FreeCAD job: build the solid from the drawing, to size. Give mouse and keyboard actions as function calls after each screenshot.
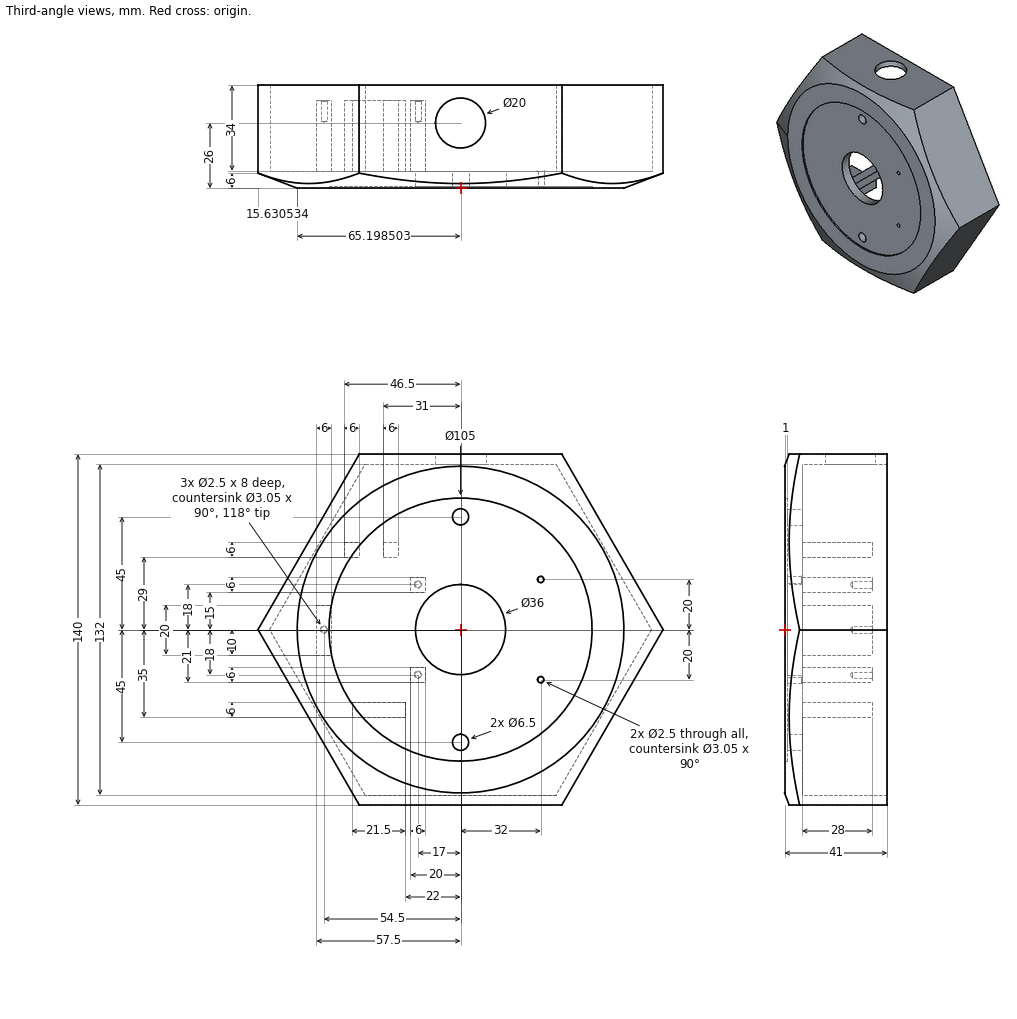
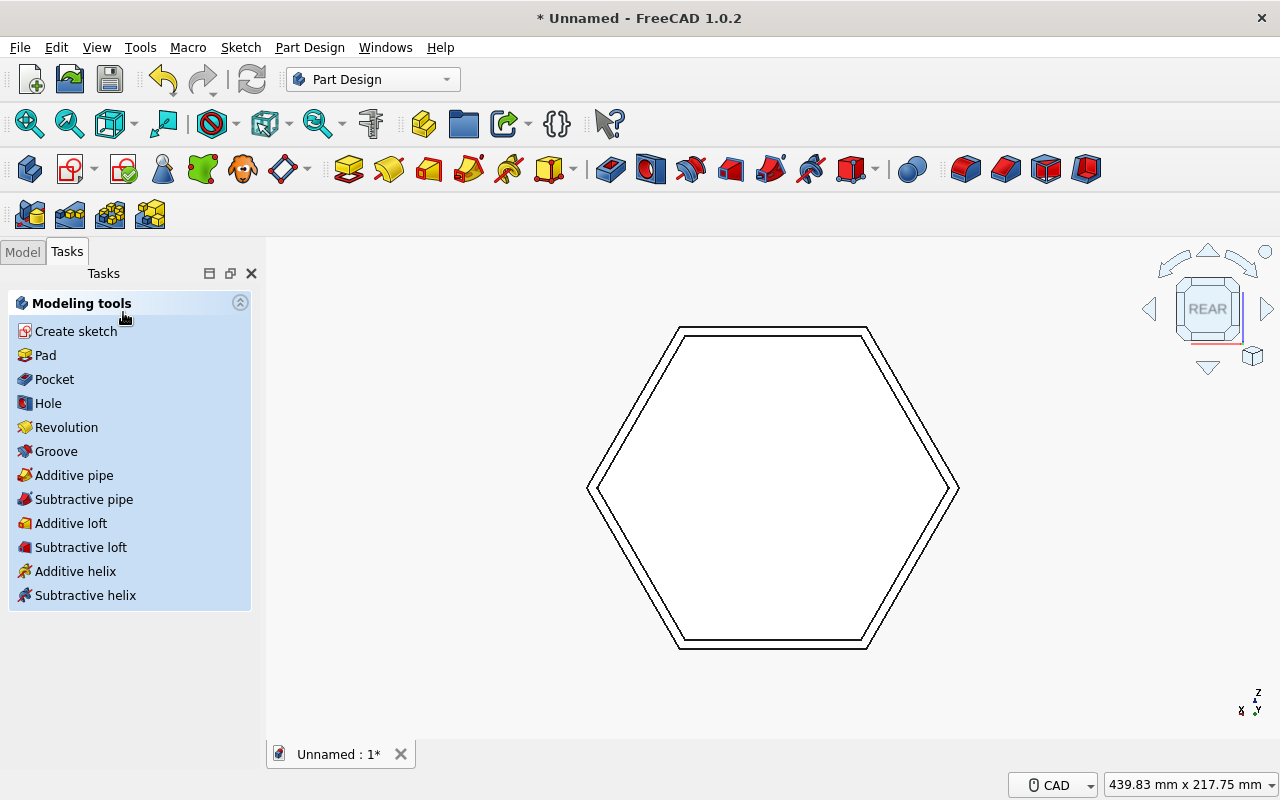
click(612, 170)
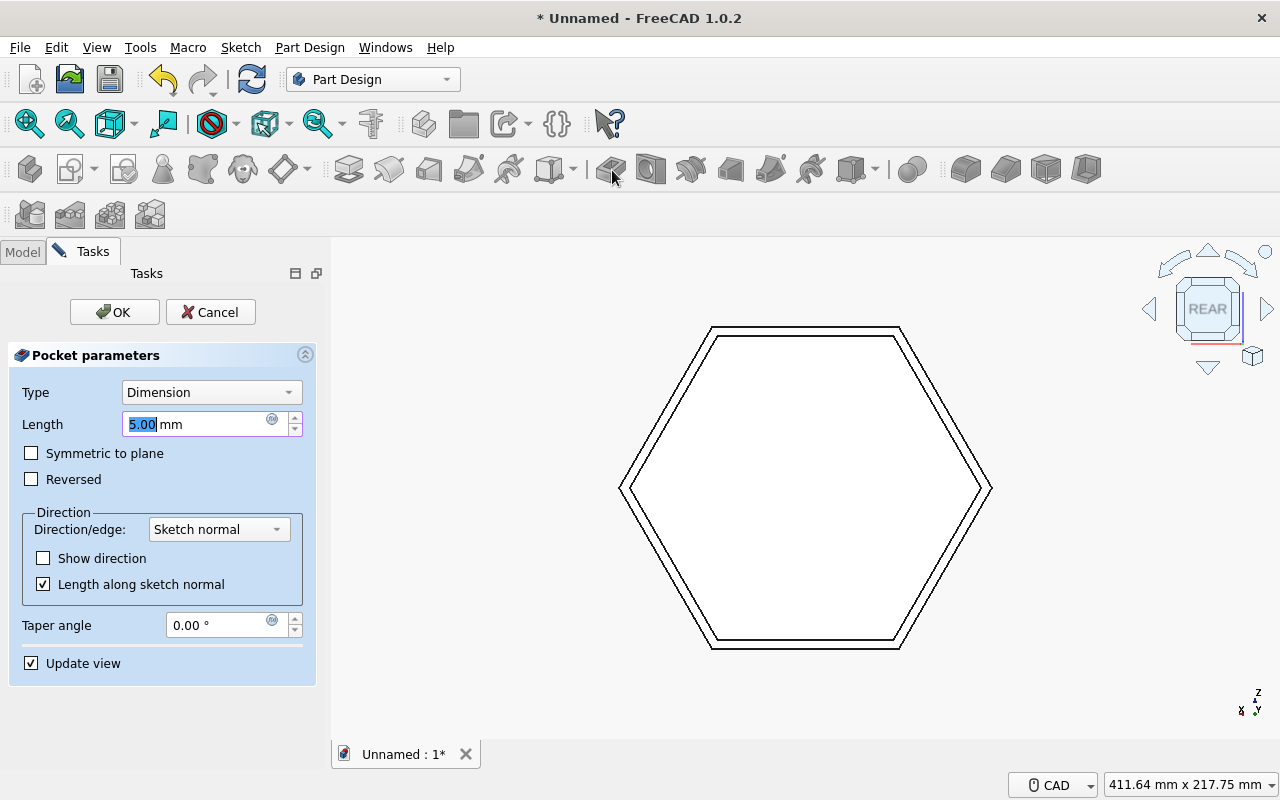
text(1)
key(Tab)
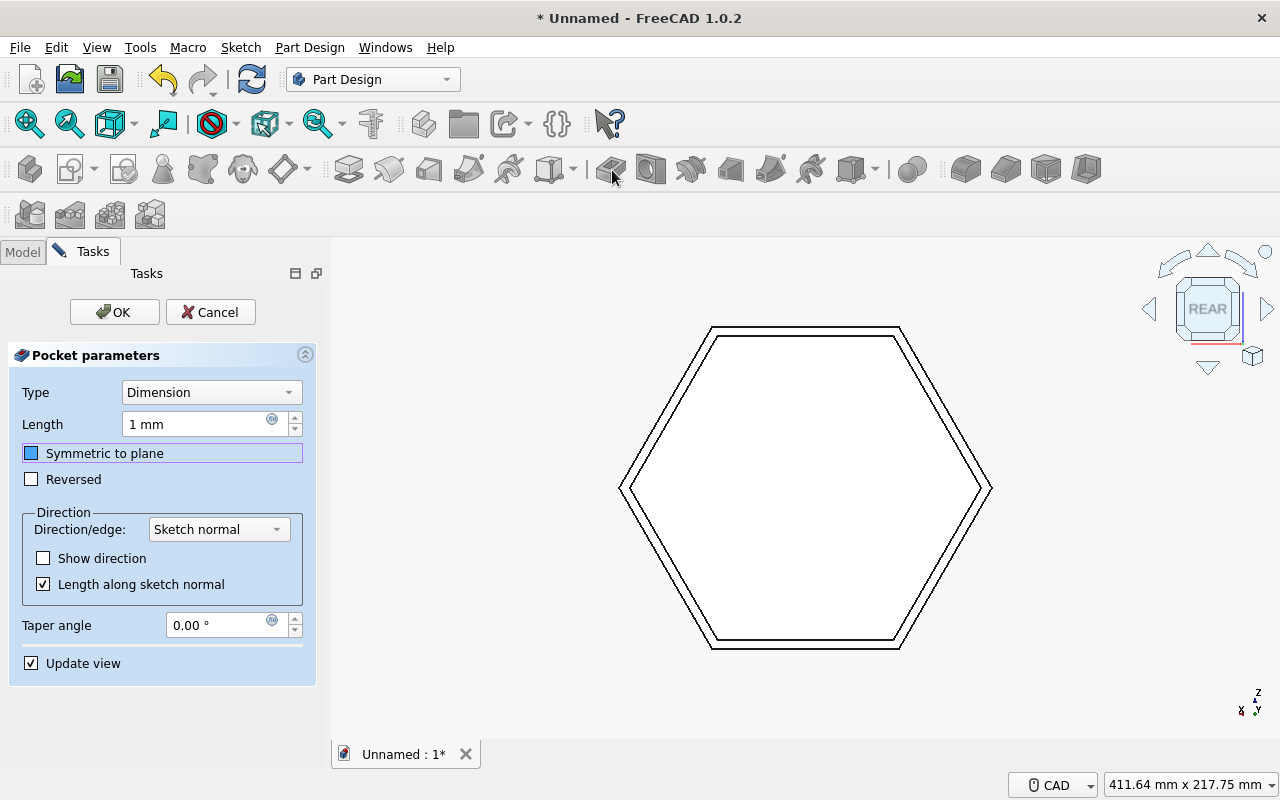
click(115, 312)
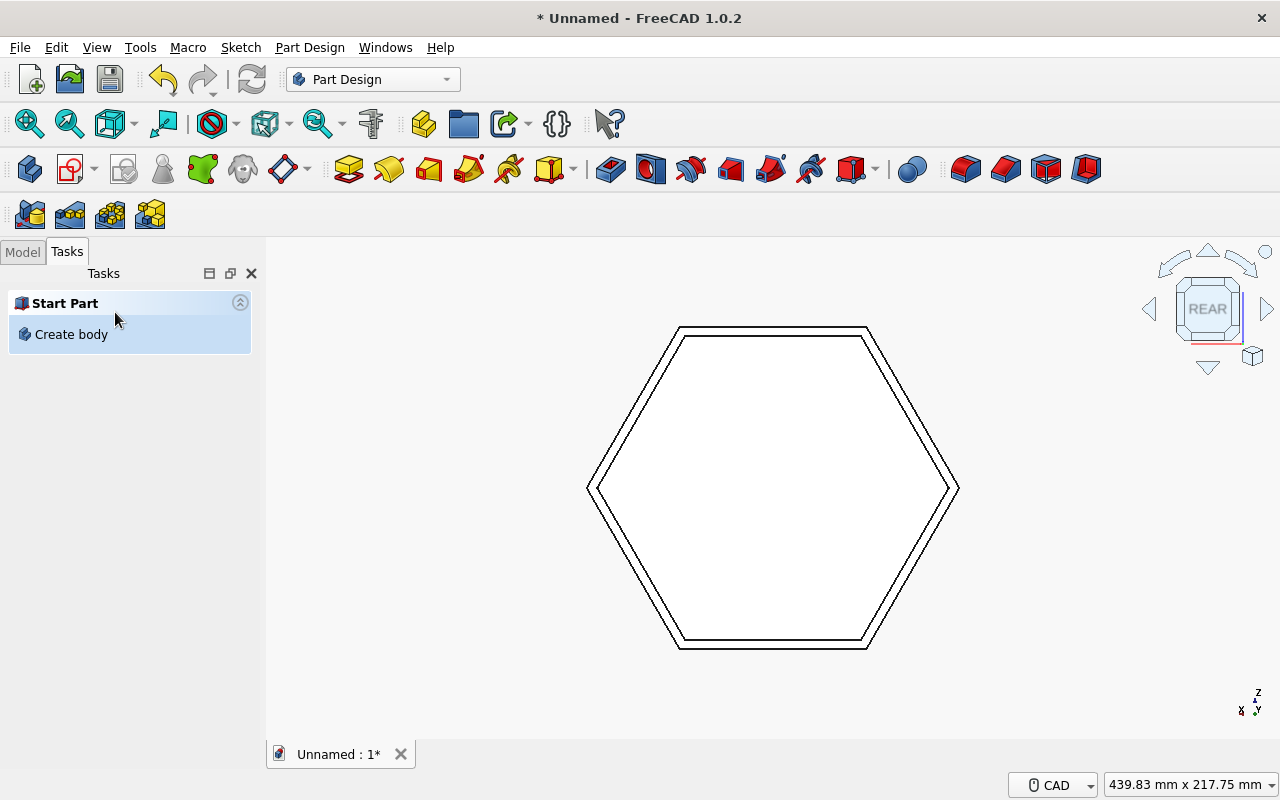
click(773, 487)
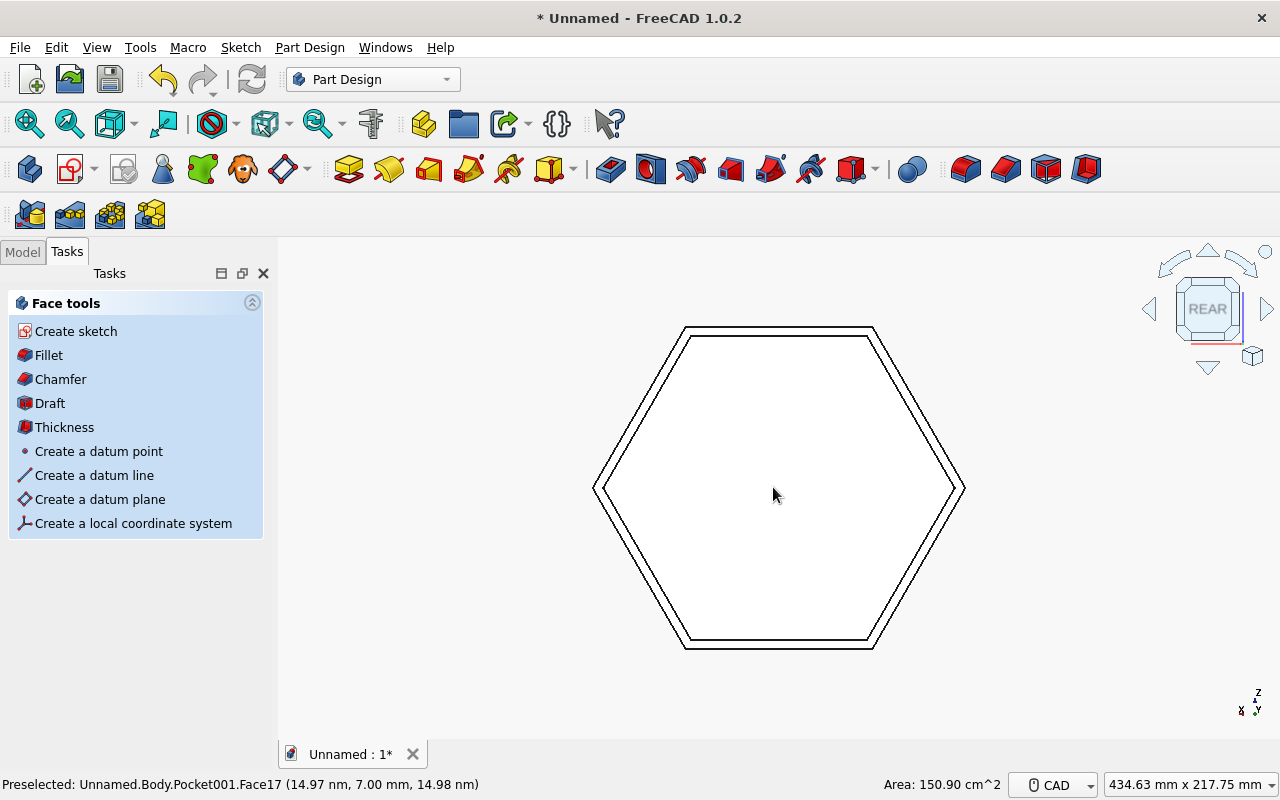
click(70, 170)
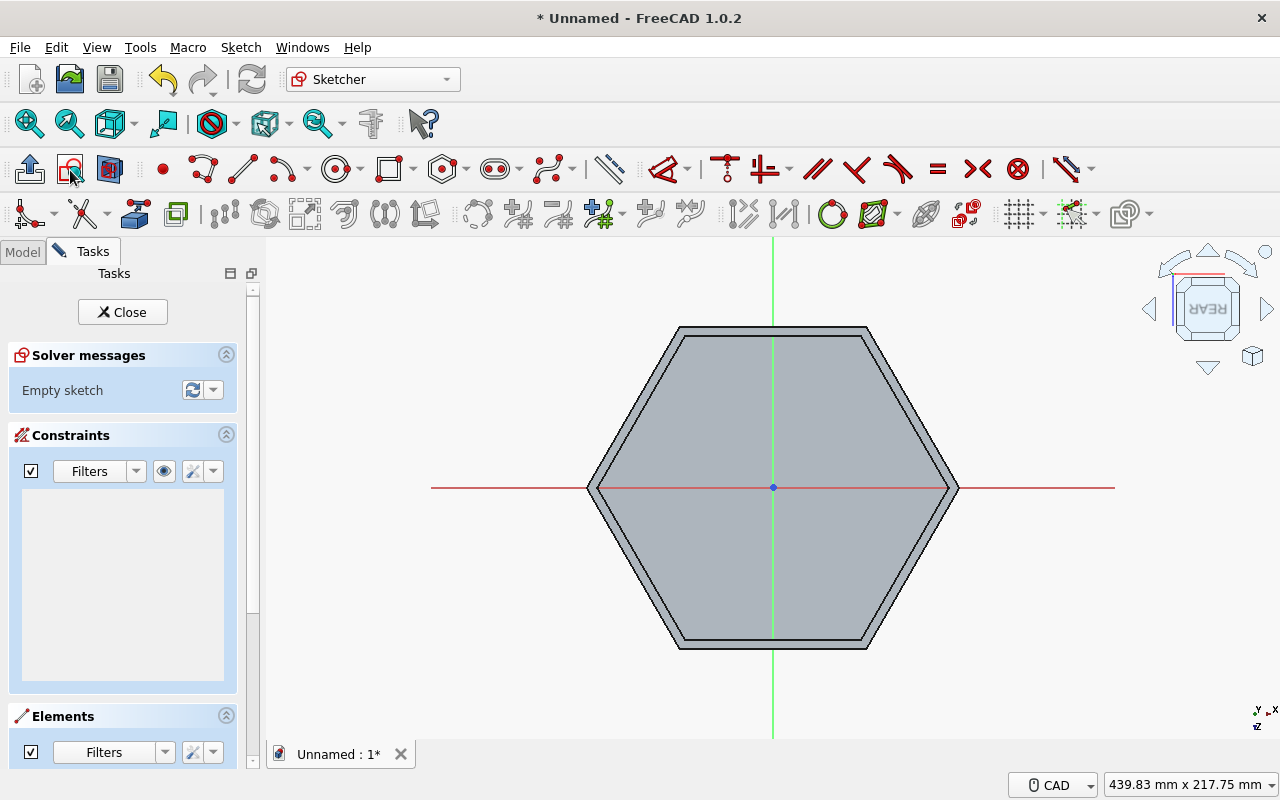
click(110, 170)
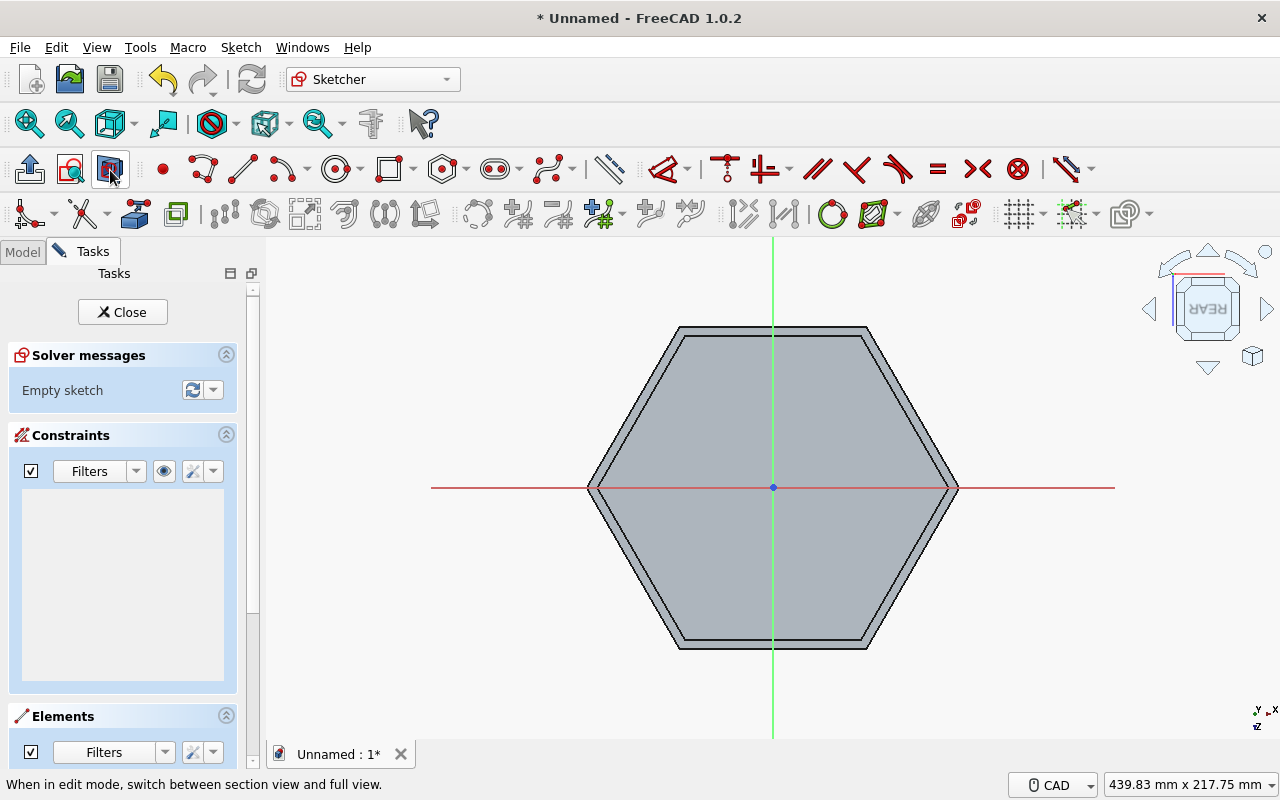
scroll(709, 488, up, 3)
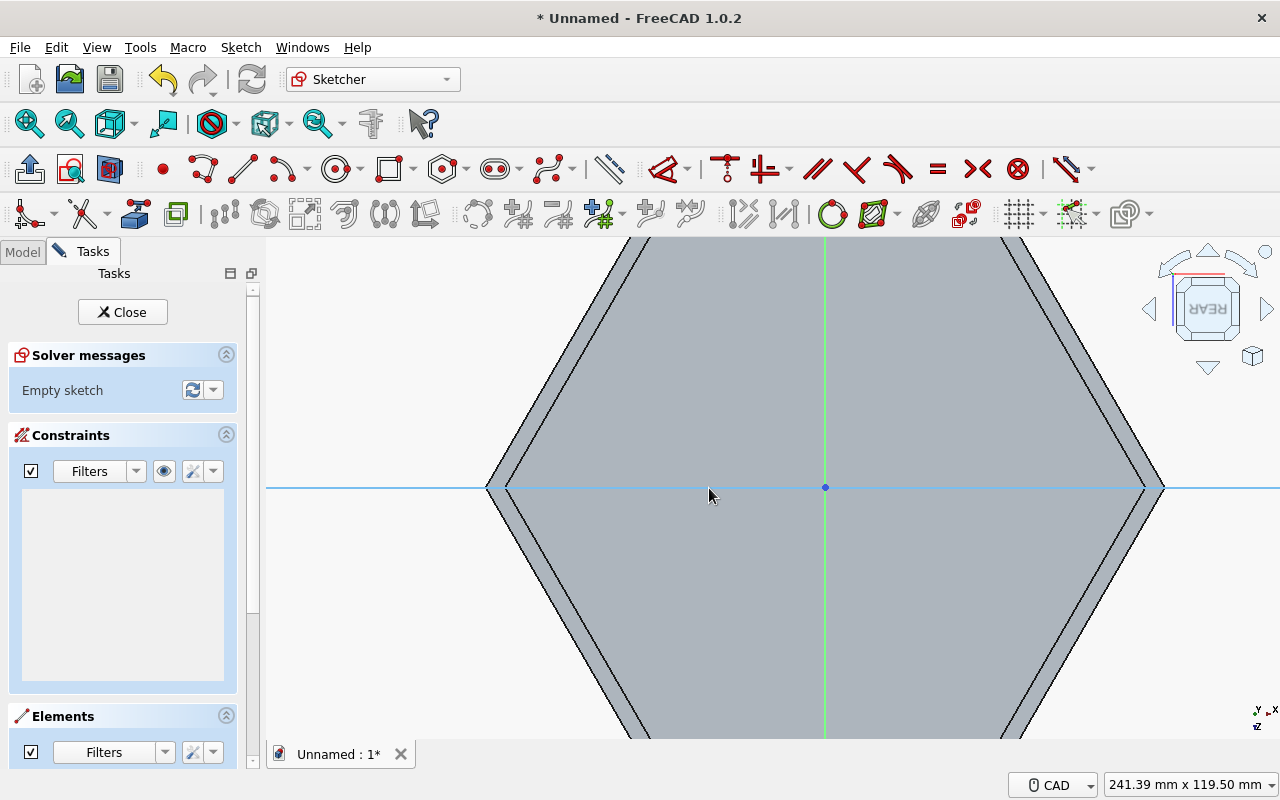
key(g)
key(r)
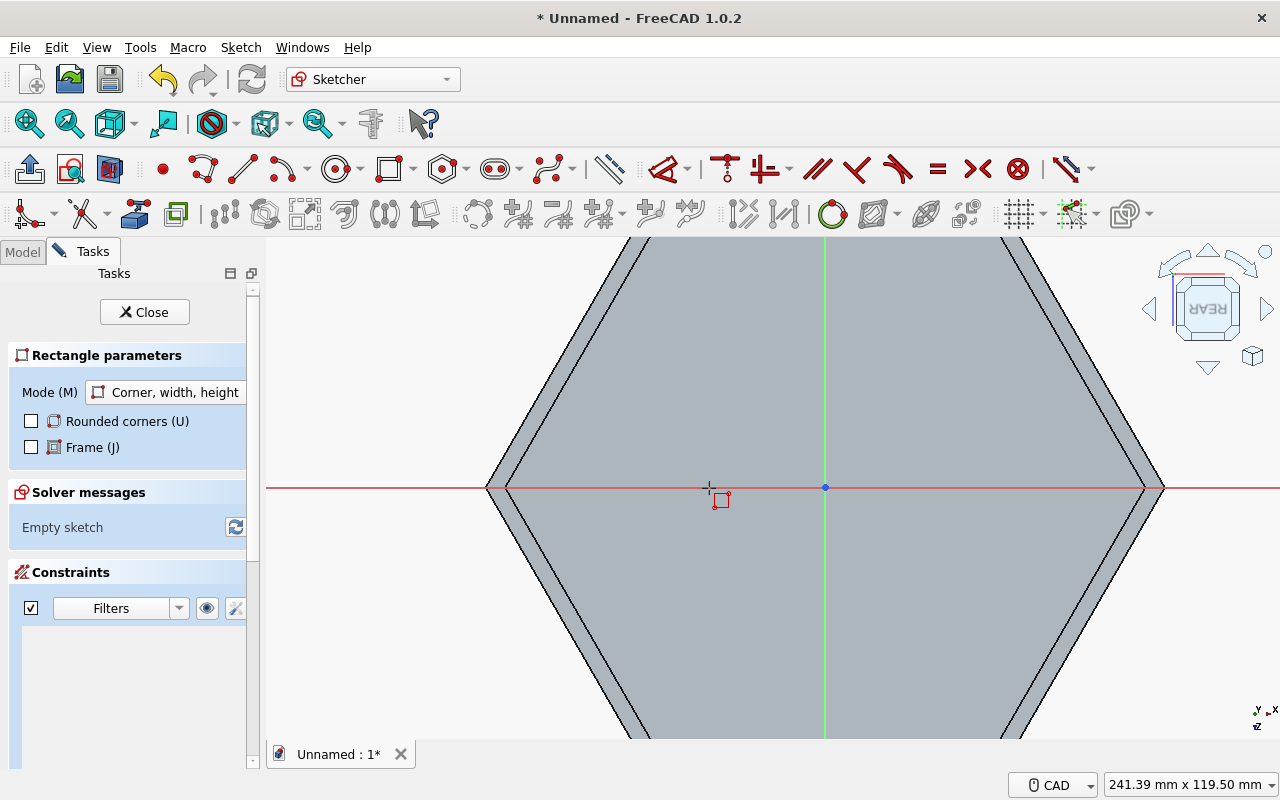
click(643, 341)
move(733, 366)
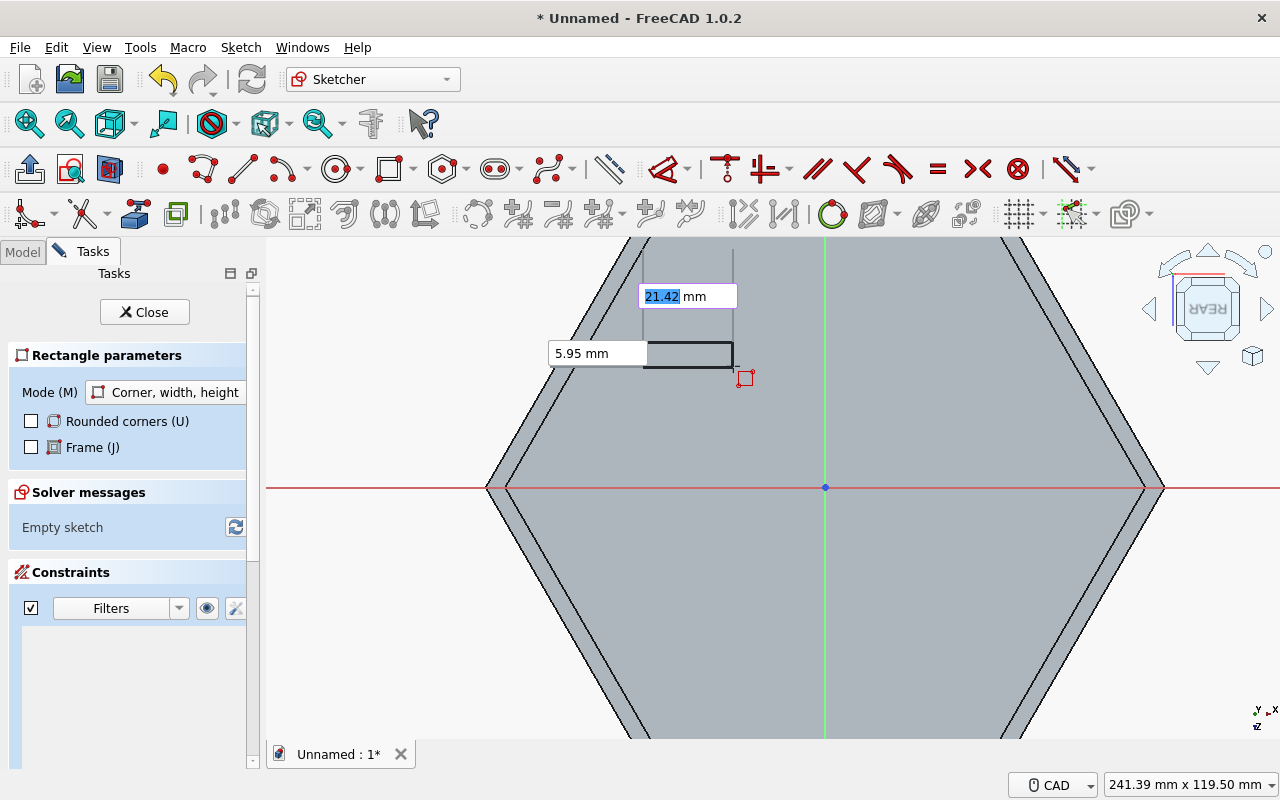
text(21.5)
key(Tab)
text(6)
key(Return)